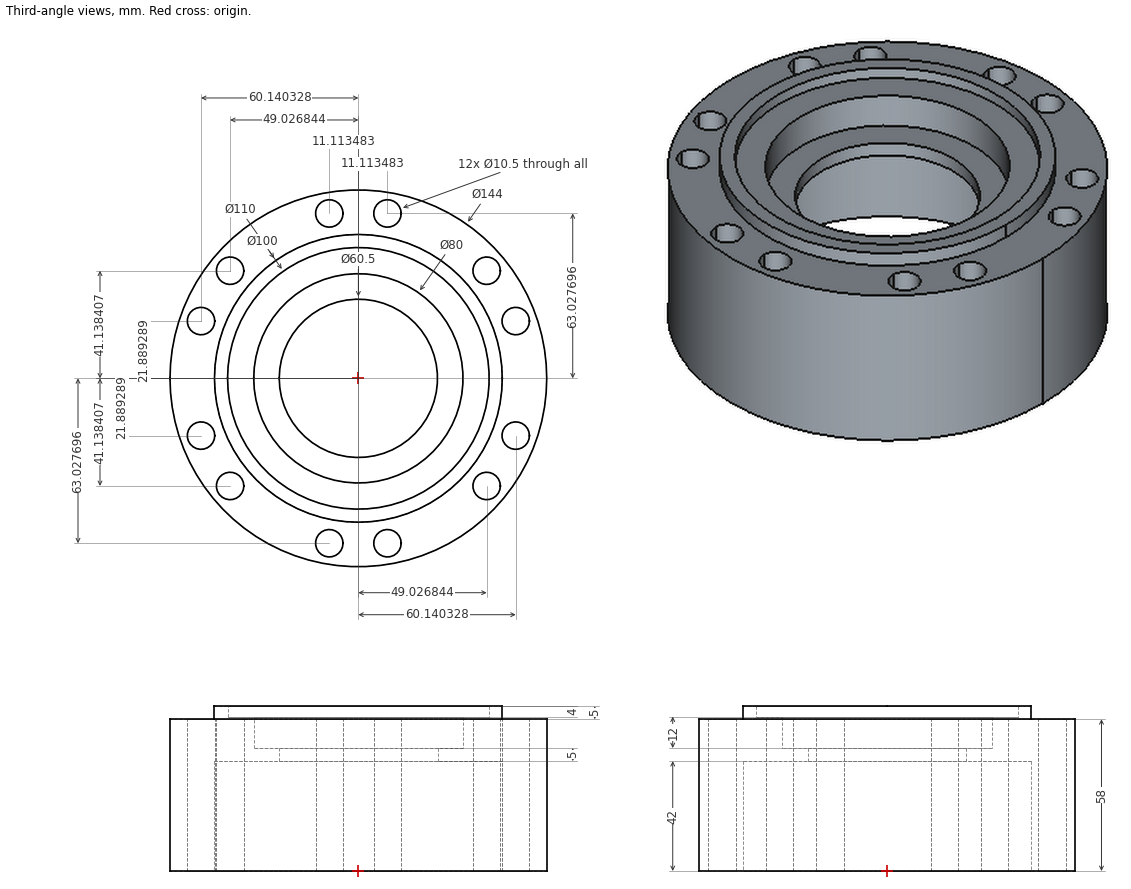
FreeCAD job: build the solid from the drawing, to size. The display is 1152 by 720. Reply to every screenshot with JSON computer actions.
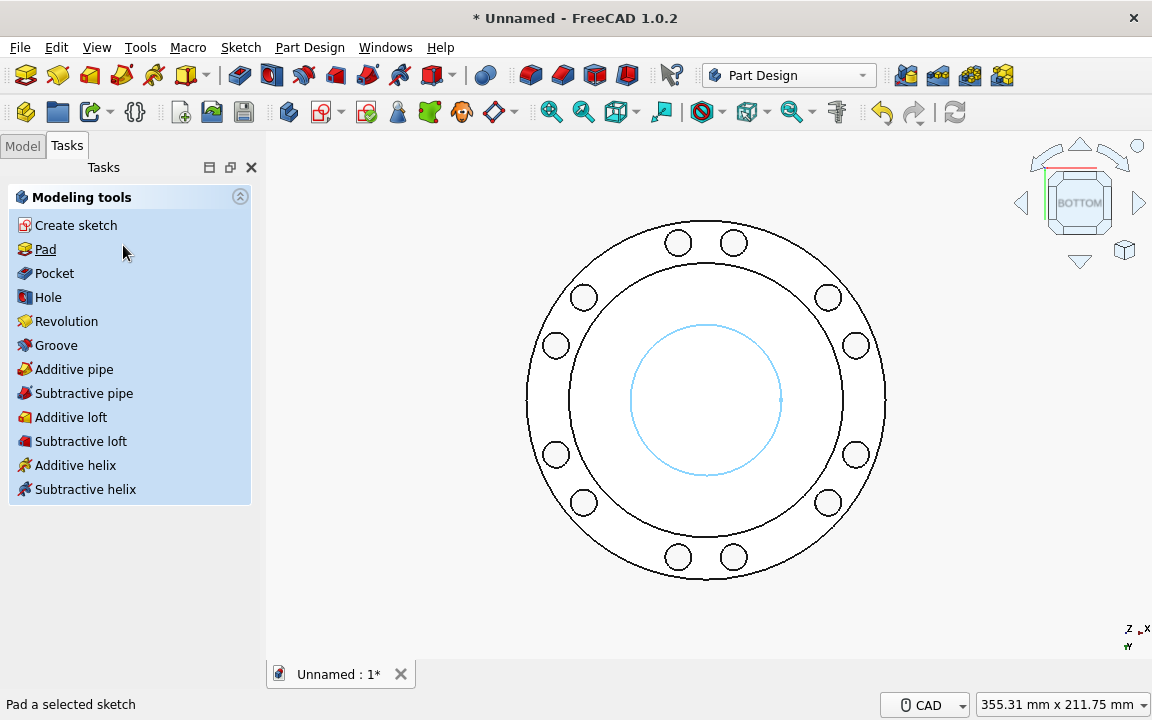
{"action": "left_click", "coordinate": [240, 76]}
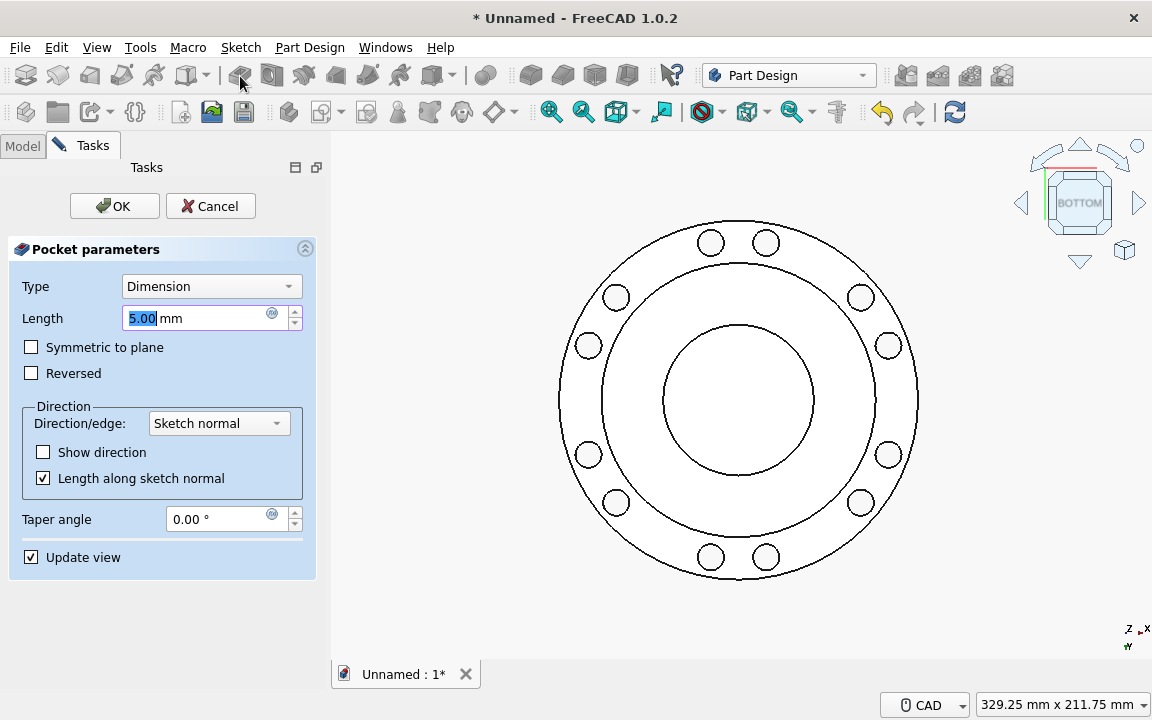
{"action": "type", "text": "5"}
{"action": "key", "text": "Tab"}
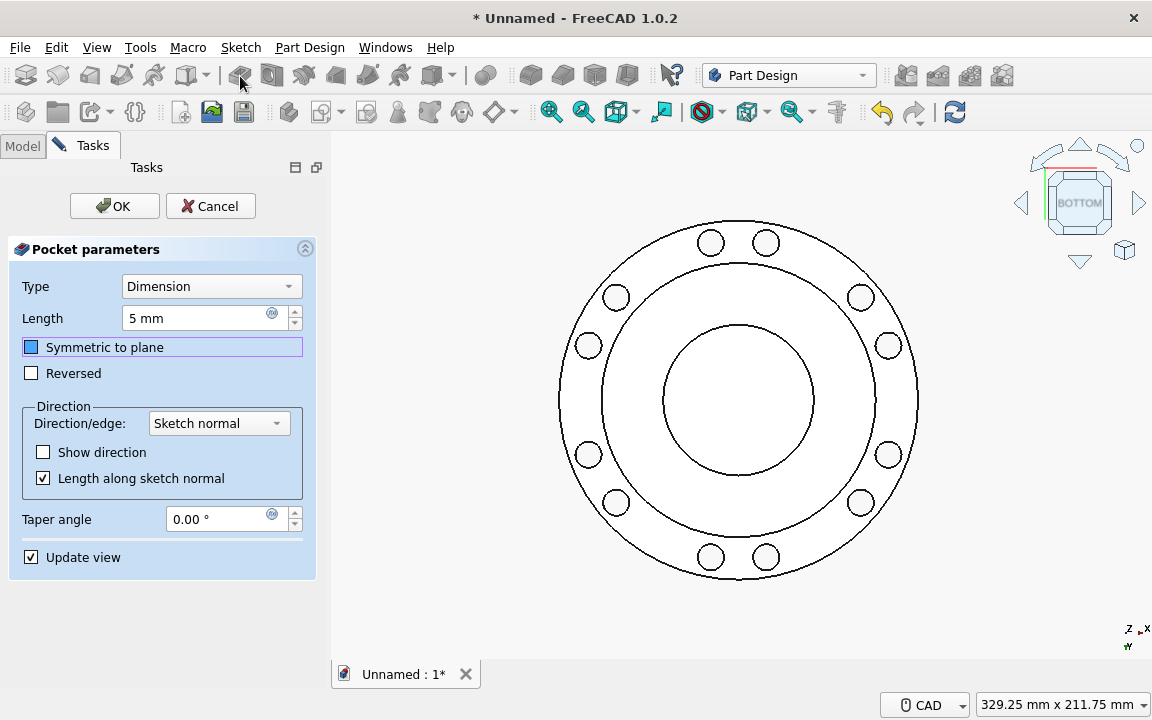
{"action": "left_click", "coordinate": [115, 206]}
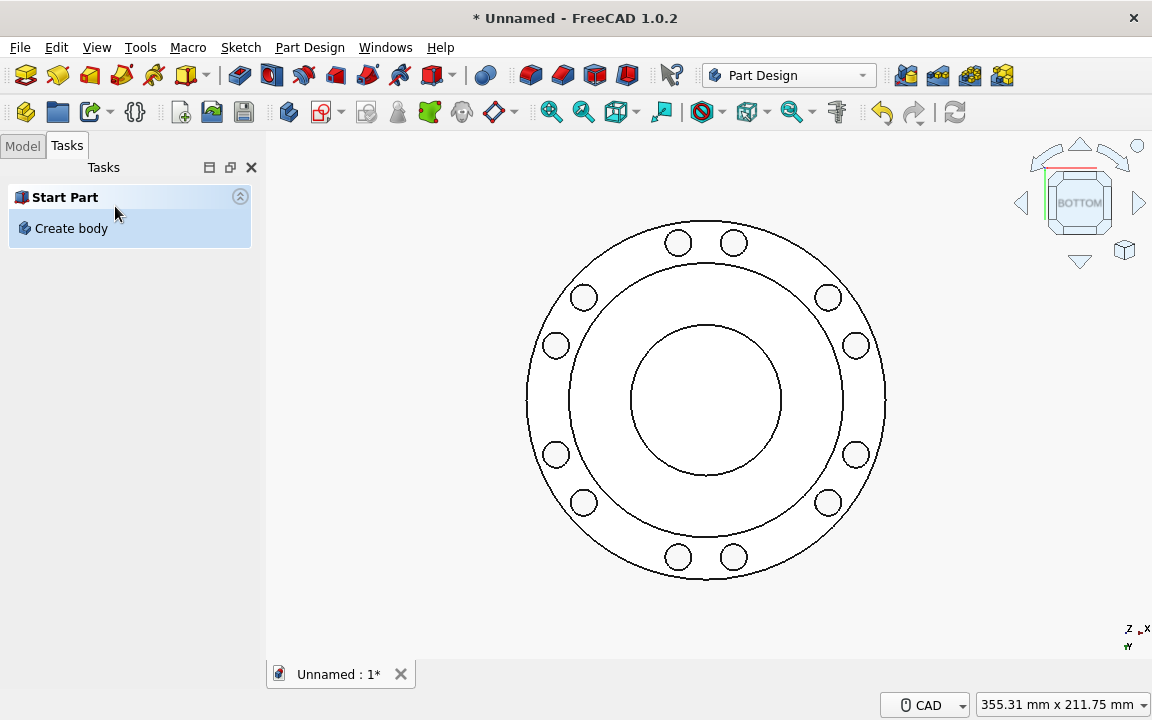
{"action": "left_click", "coordinate": [706, 399]}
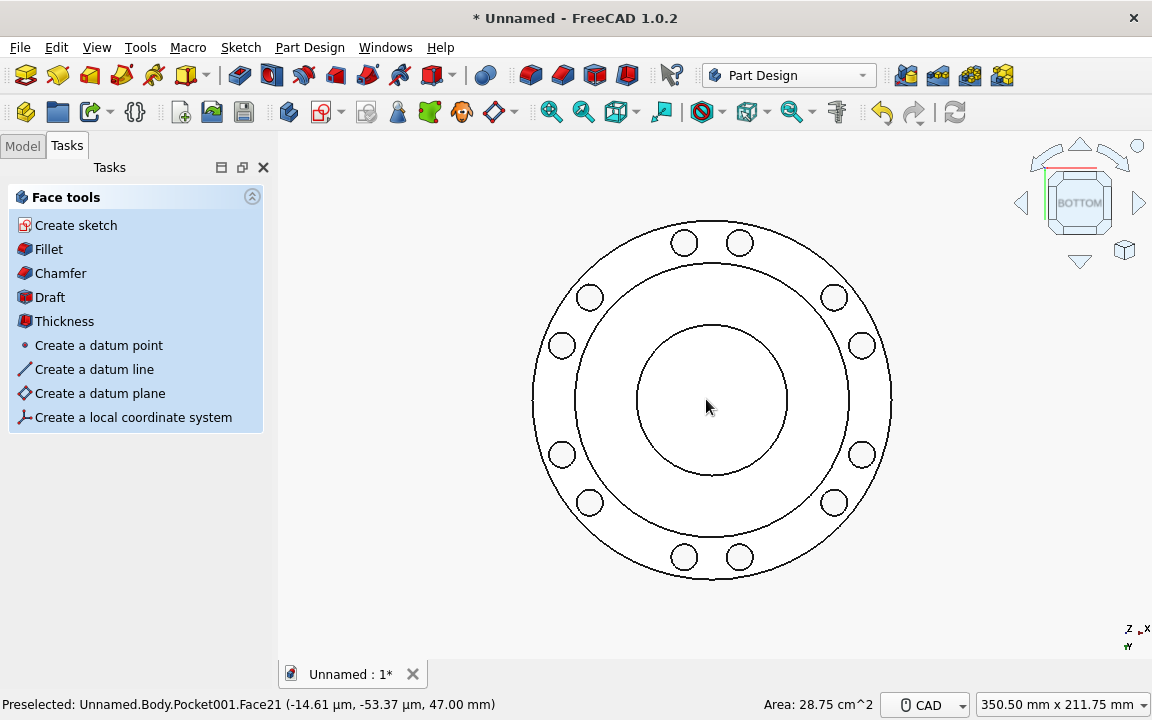
{"action": "left_click", "coordinate": [322, 112]}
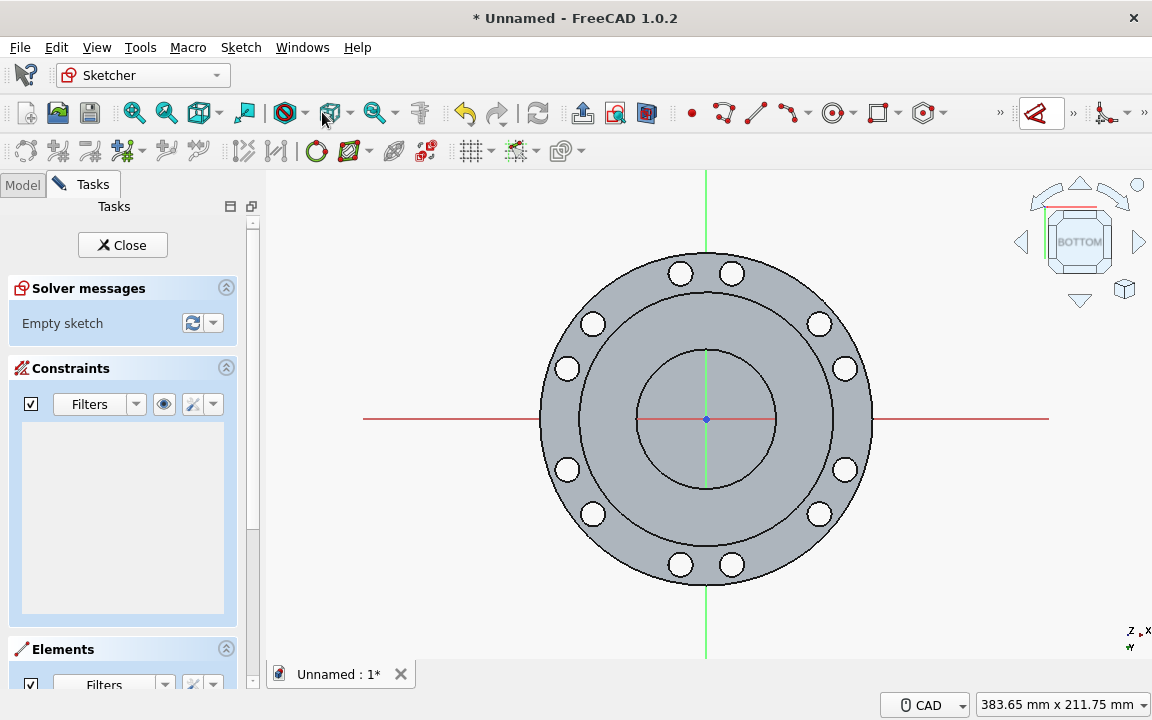
{"action": "key", "text": "q s"}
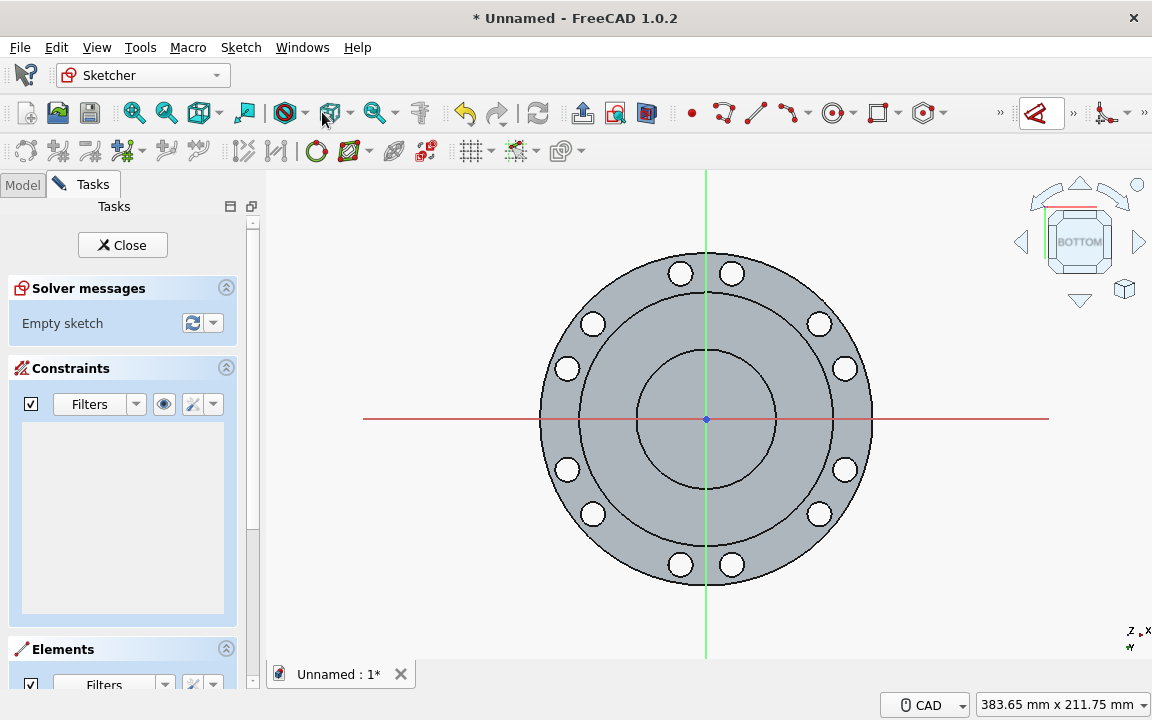
{"action": "scroll", "coordinate": [786, 425], "scroll_direction": "up", "scroll_amount": 3}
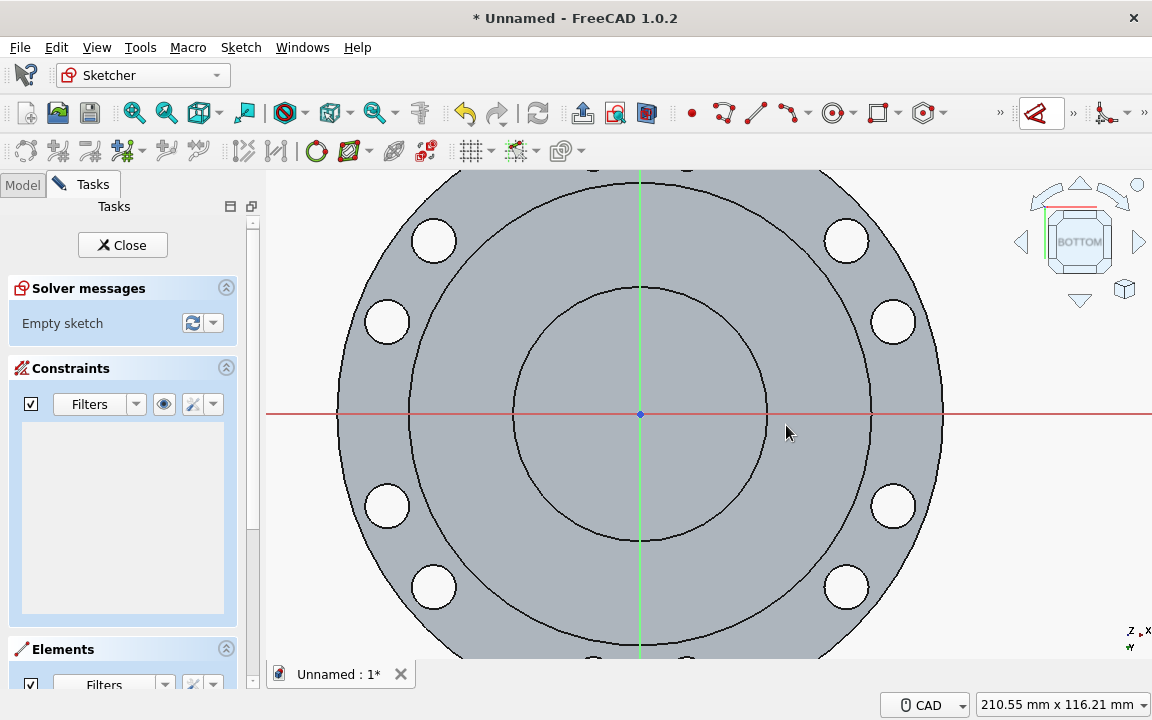
{"action": "key", "text": "g c"}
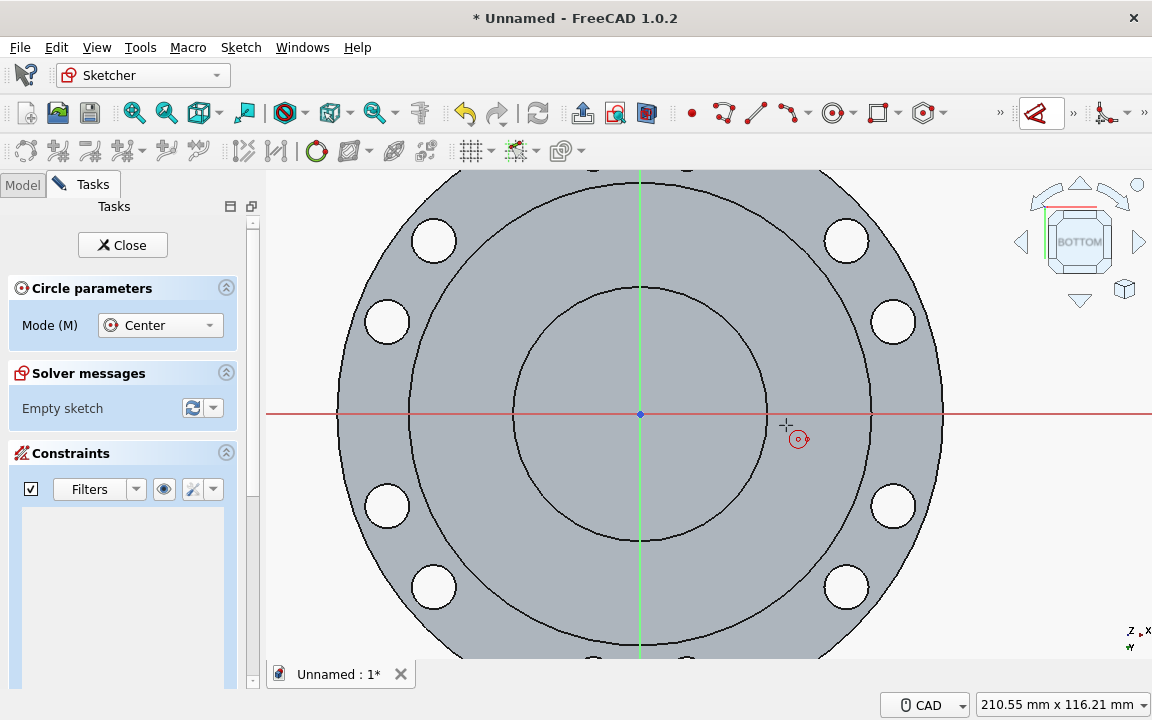
{"action": "left_click", "coordinate": [640, 414]}
{"action": "left_click", "coordinate": [759, 295]}
{"action": "key", "text": "Escape"}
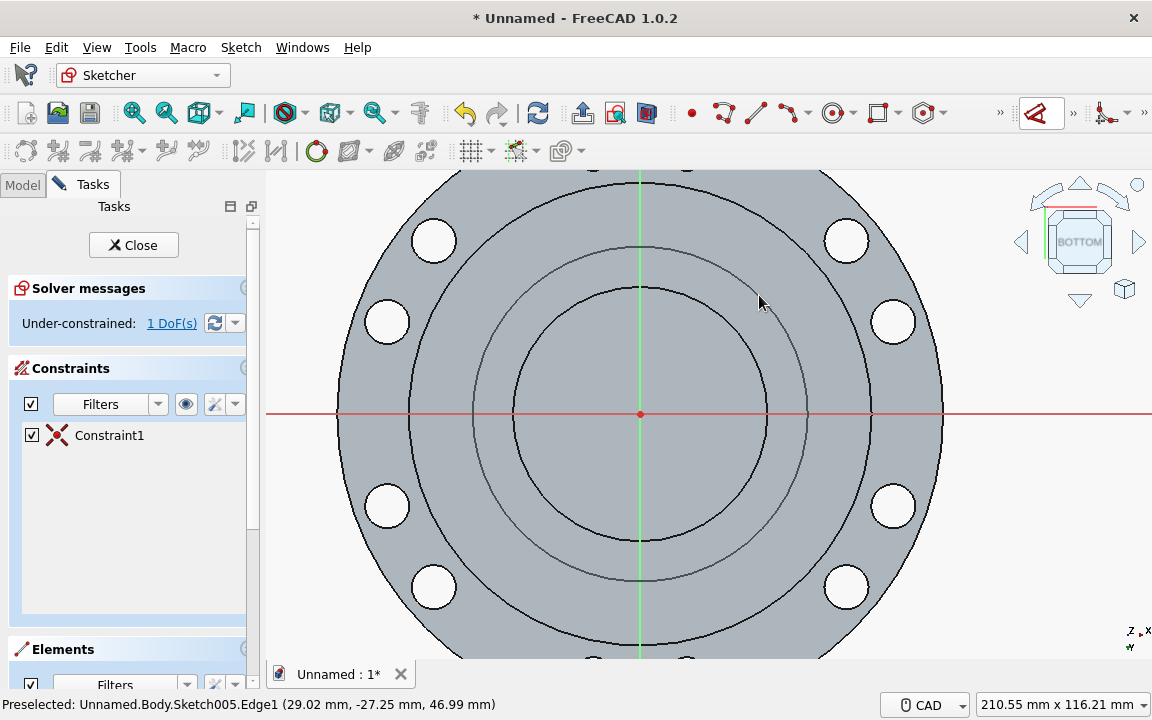
{"action": "left_click", "coordinate": [1036, 114]}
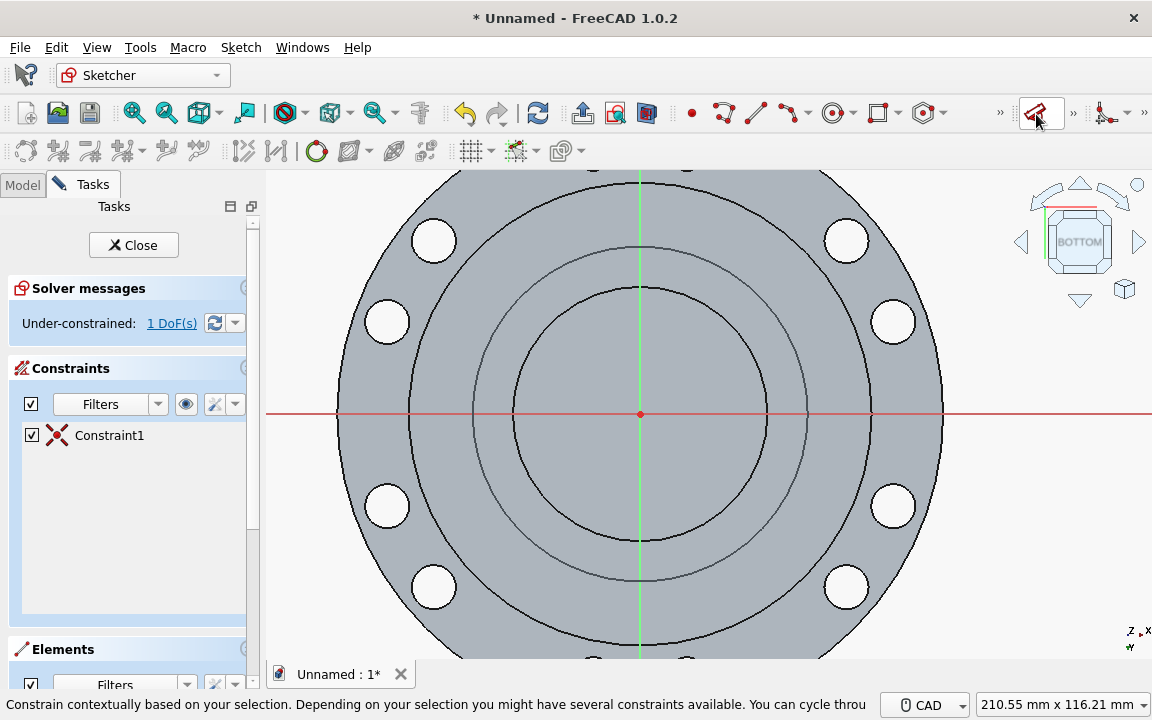
{"action": "left_click", "coordinate": [758, 295]}
{"action": "left_click", "coordinate": [781, 272]}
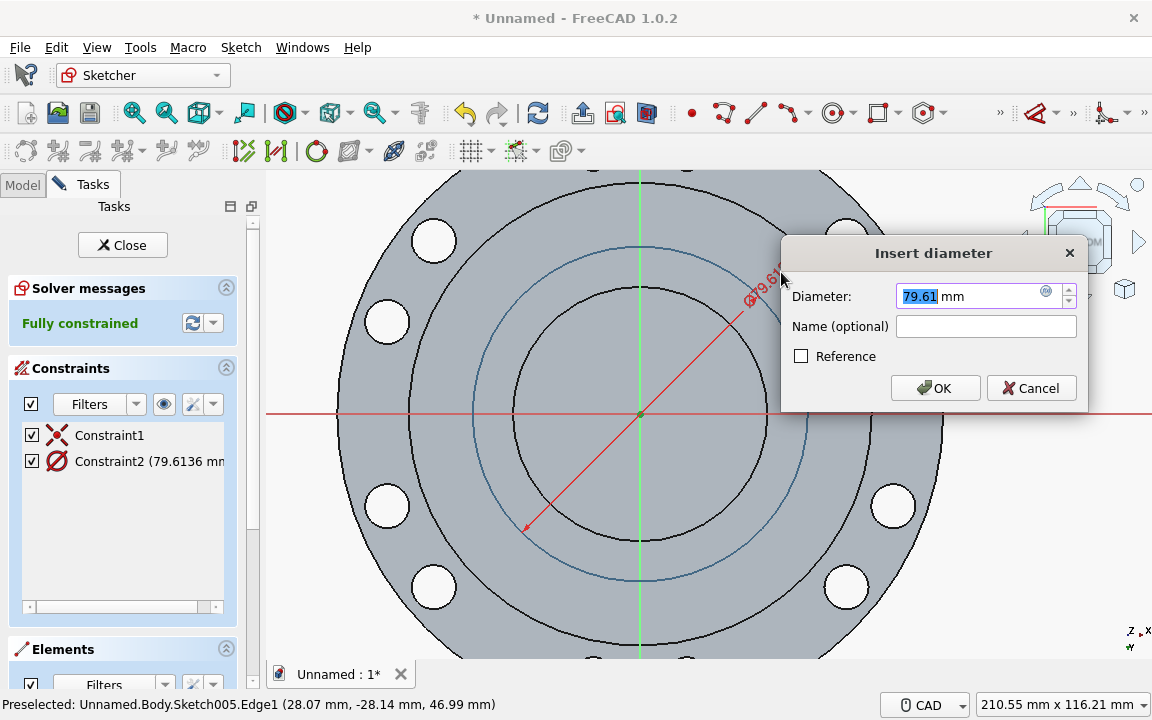
{"action": "type", "text": "80"}
{"action": "key", "text": "Return"}
{"action": "key", "text": "Escape"}